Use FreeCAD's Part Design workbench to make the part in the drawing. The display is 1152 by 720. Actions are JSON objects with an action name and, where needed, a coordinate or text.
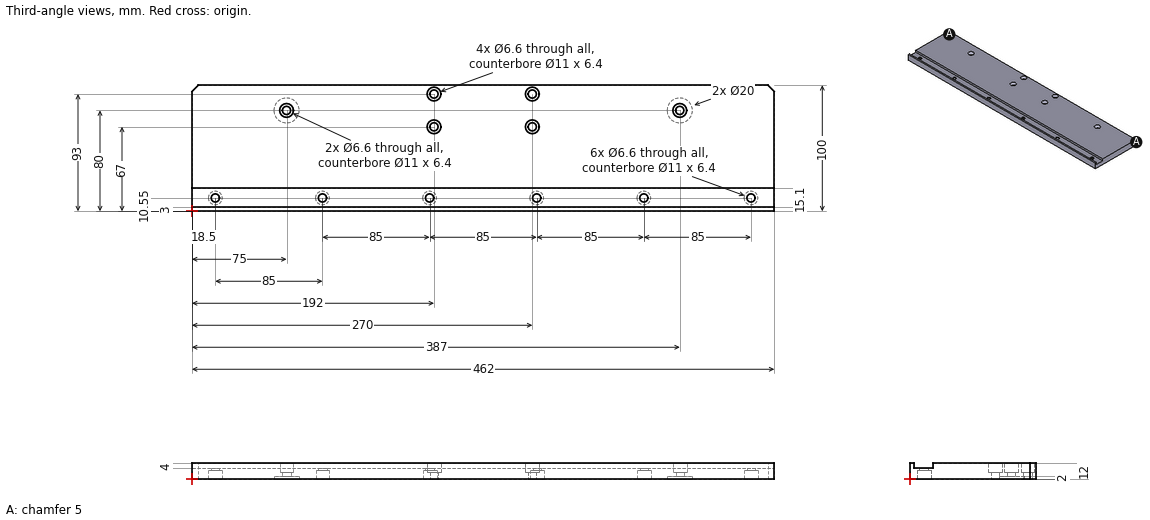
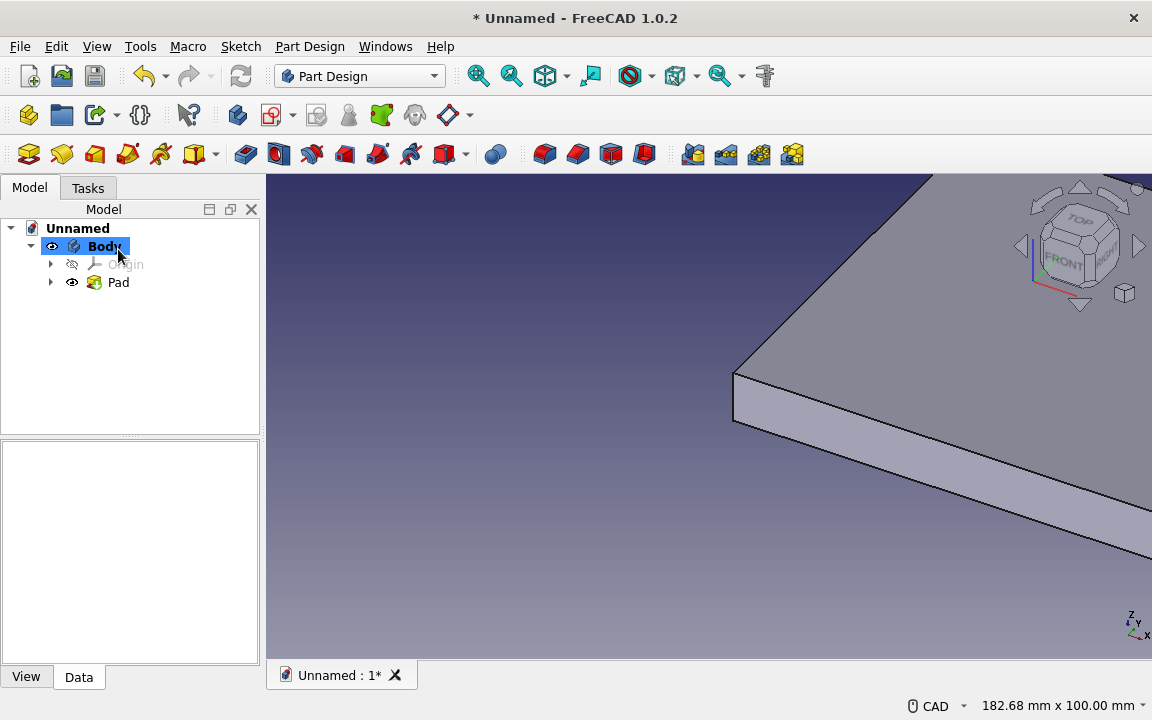
{"action": "key", "text": "v f"}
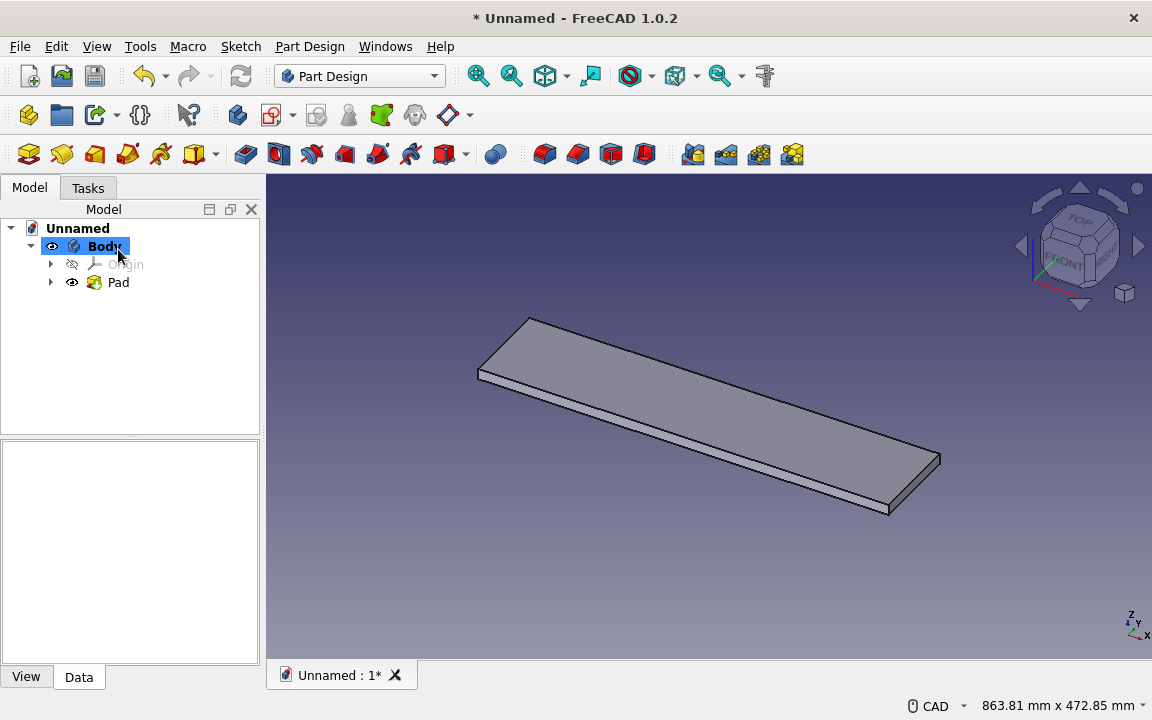
{"action": "left_click", "coordinate": [826, 449]}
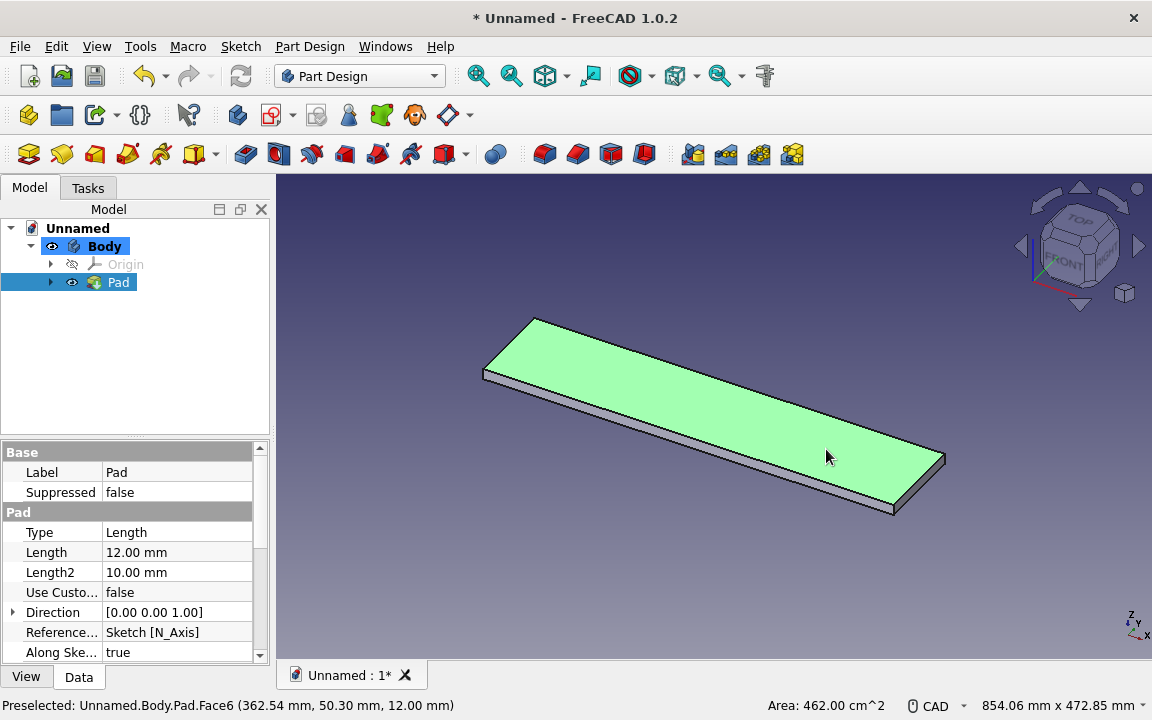
{"action": "left_click", "coordinate": [270, 116]}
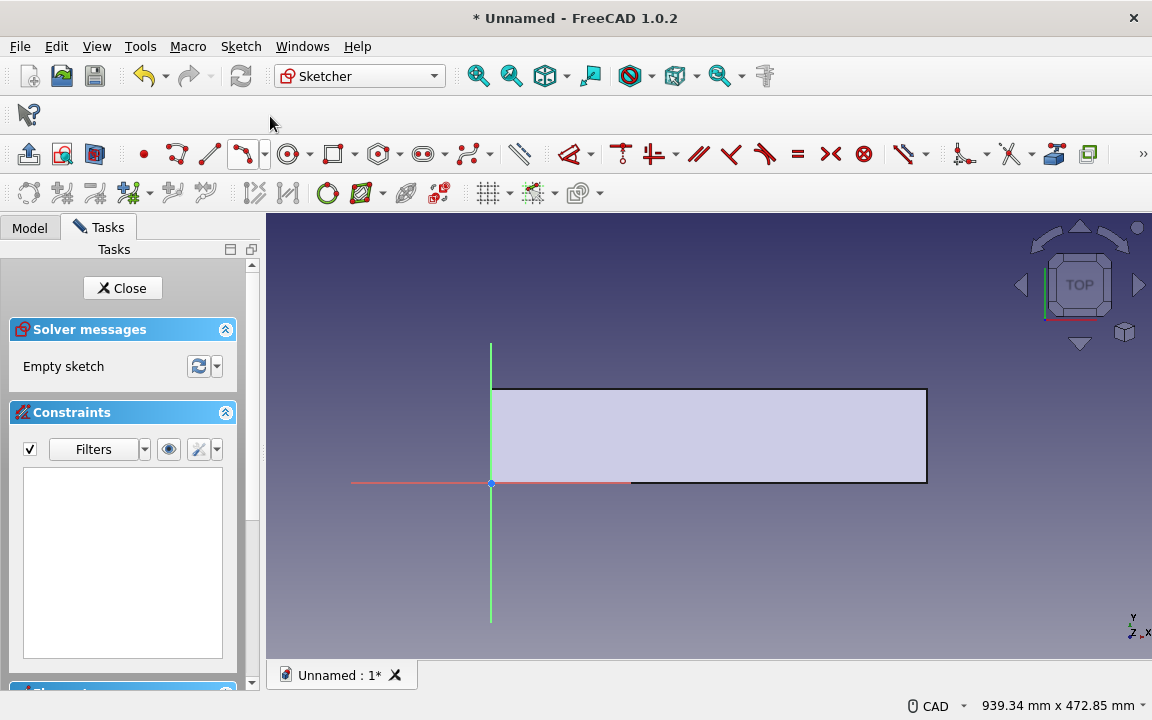
{"action": "left_click", "coordinate": [332, 154]}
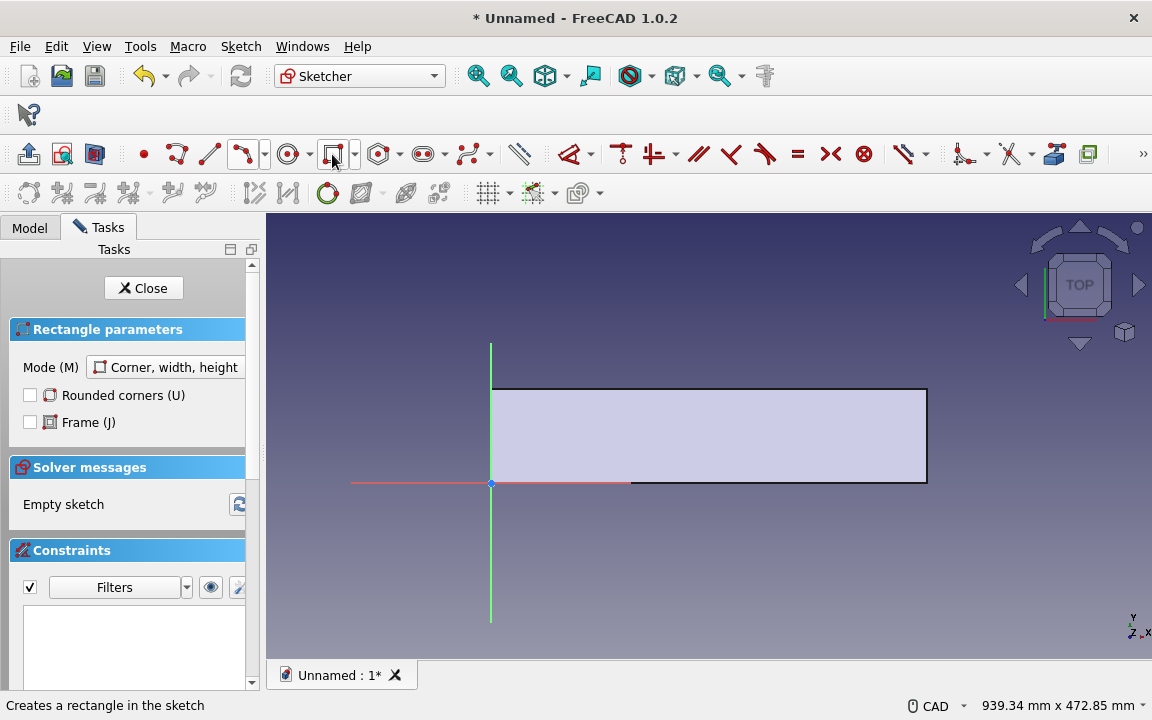
{"action": "left_click", "coordinate": [491, 466]}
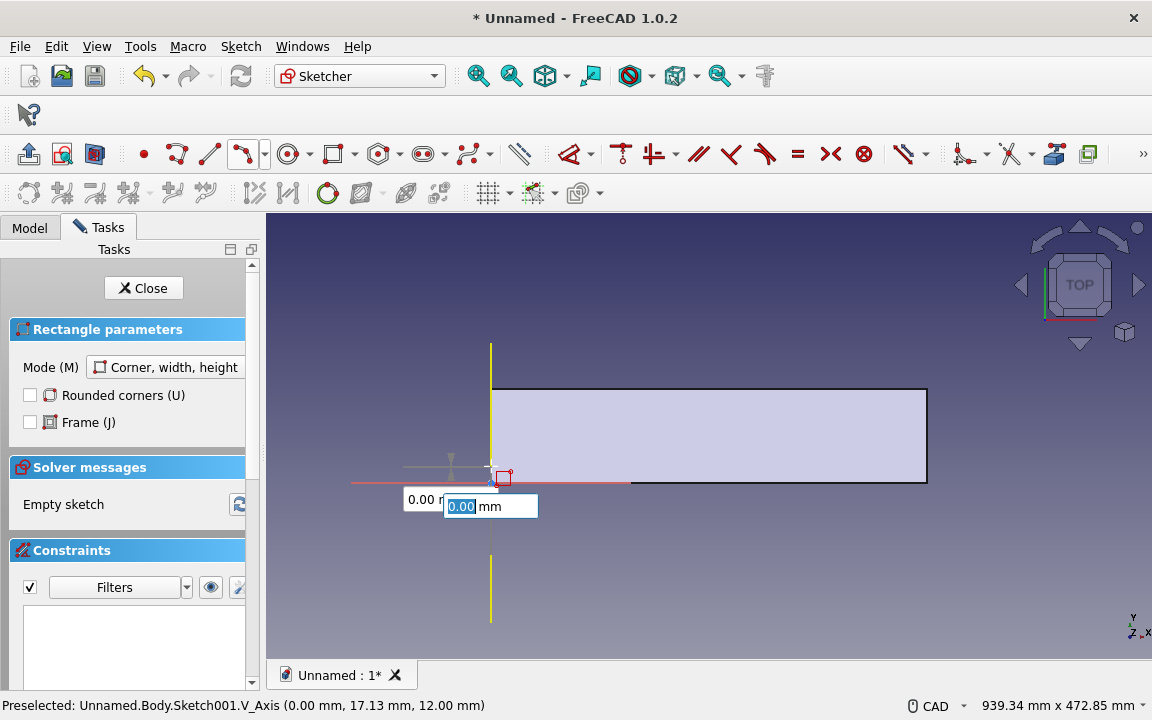
{"action": "scroll", "coordinate": [927, 480], "scroll_direction": "up", "scroll_amount": 9}
{"action": "mouse_move", "coordinate": [923, 479]}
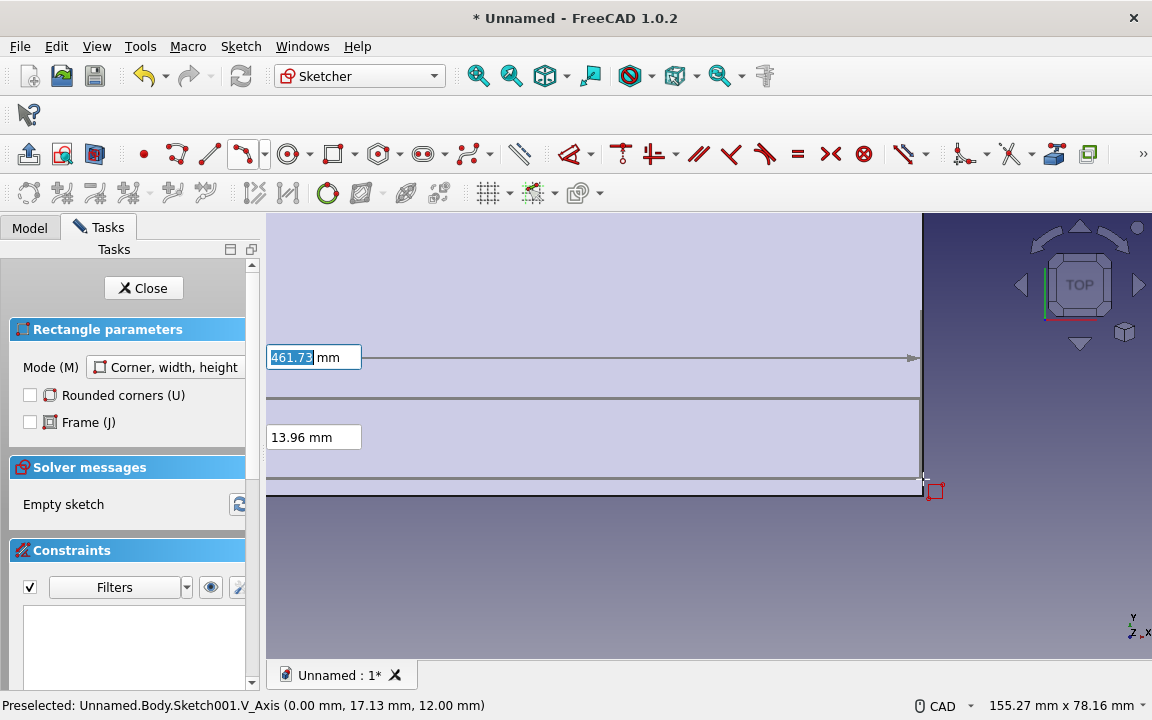
{"action": "type", "text": "462"}
{"action": "key", "text": "Tab"}
{"action": "type", "text": "15.1"}
{"action": "key", "text": "Return"}
{"action": "key", "text": "Escape"}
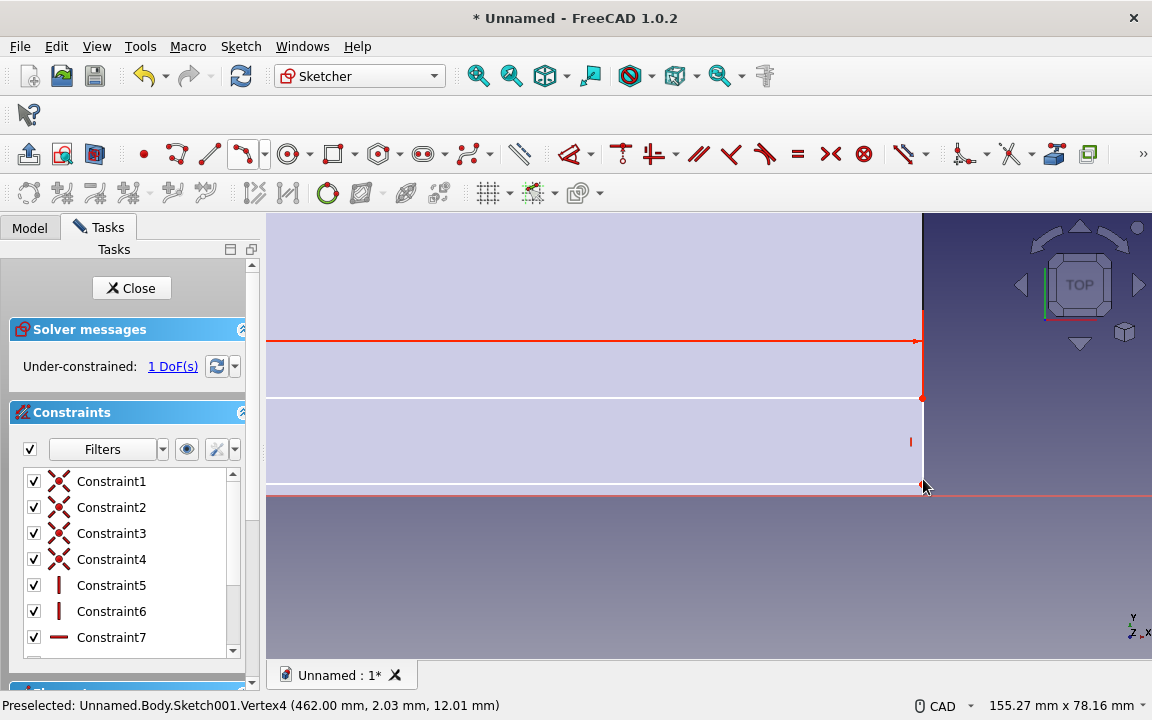
{"action": "left_click", "coordinate": [568, 154]}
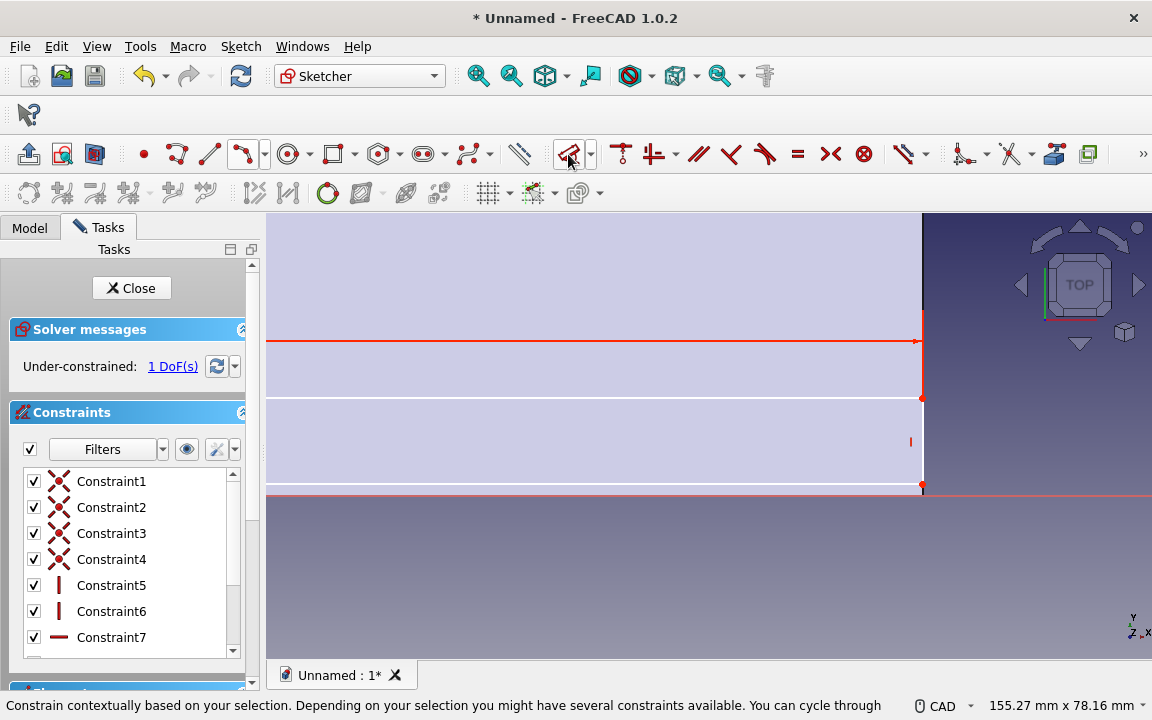
{"action": "scroll", "coordinate": [903, 434], "scroll_direction": "down", "scroll_amount": 8}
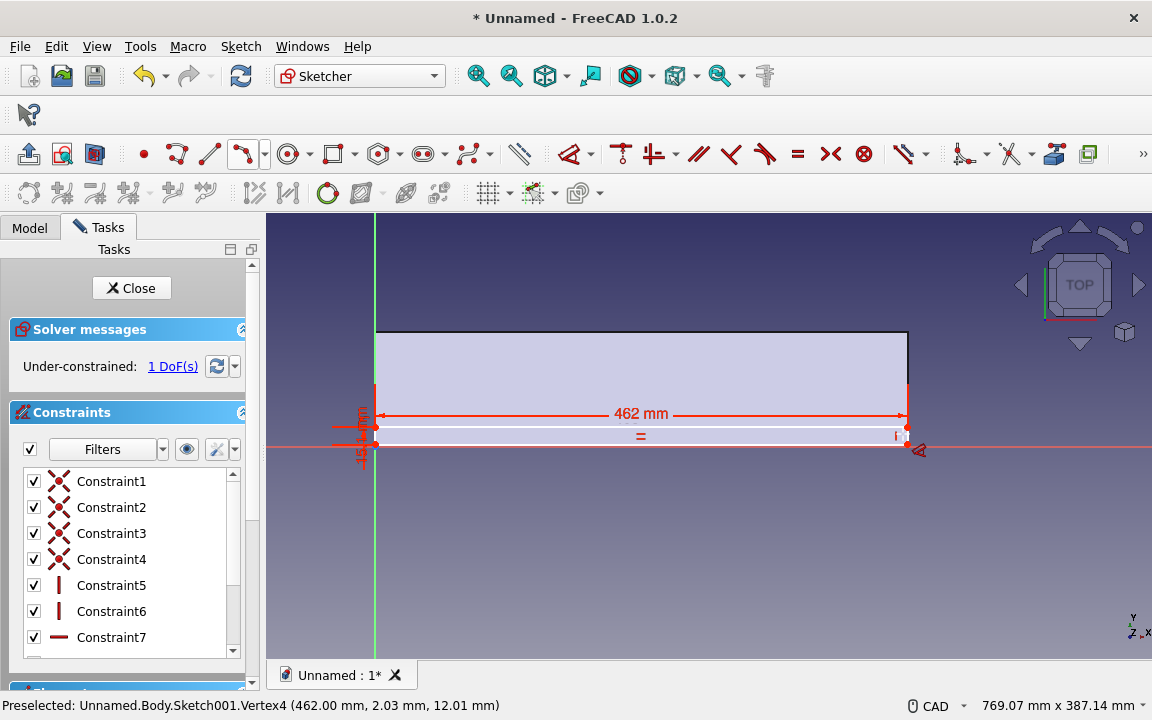
{"action": "scroll", "coordinate": [375, 445], "scroll_direction": "up", "scroll_amount": 13}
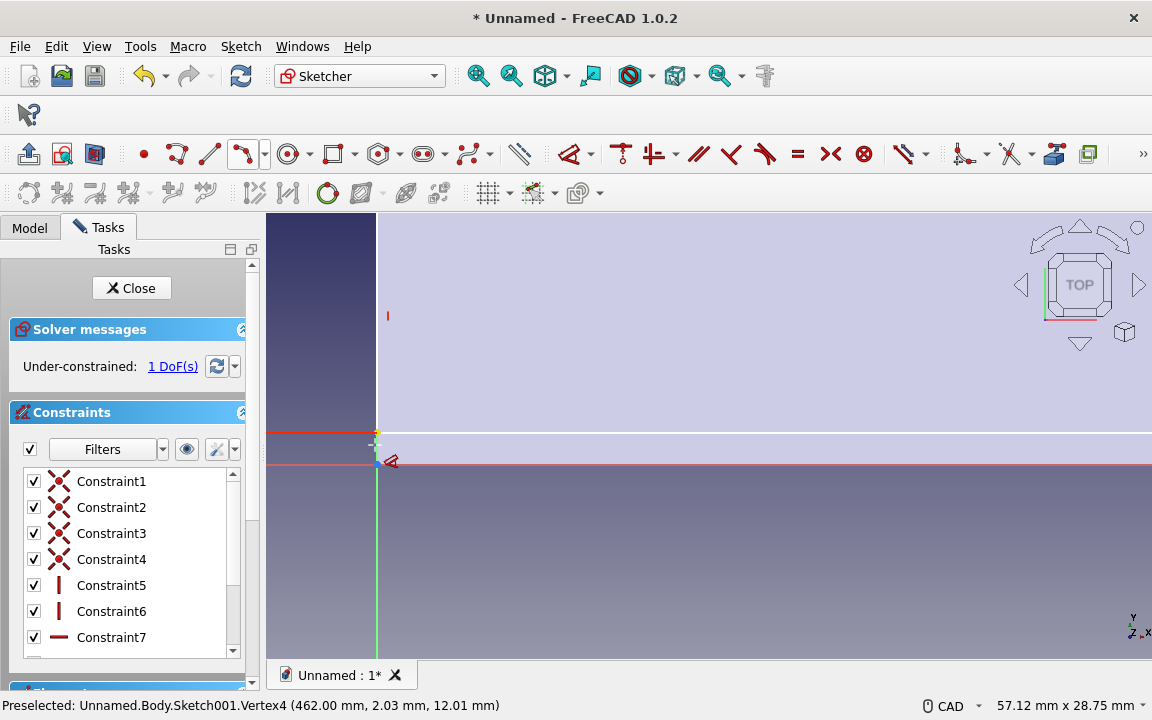
{"action": "left_click", "coordinate": [377, 433]}
{"action": "left_click", "coordinate": [343, 449]}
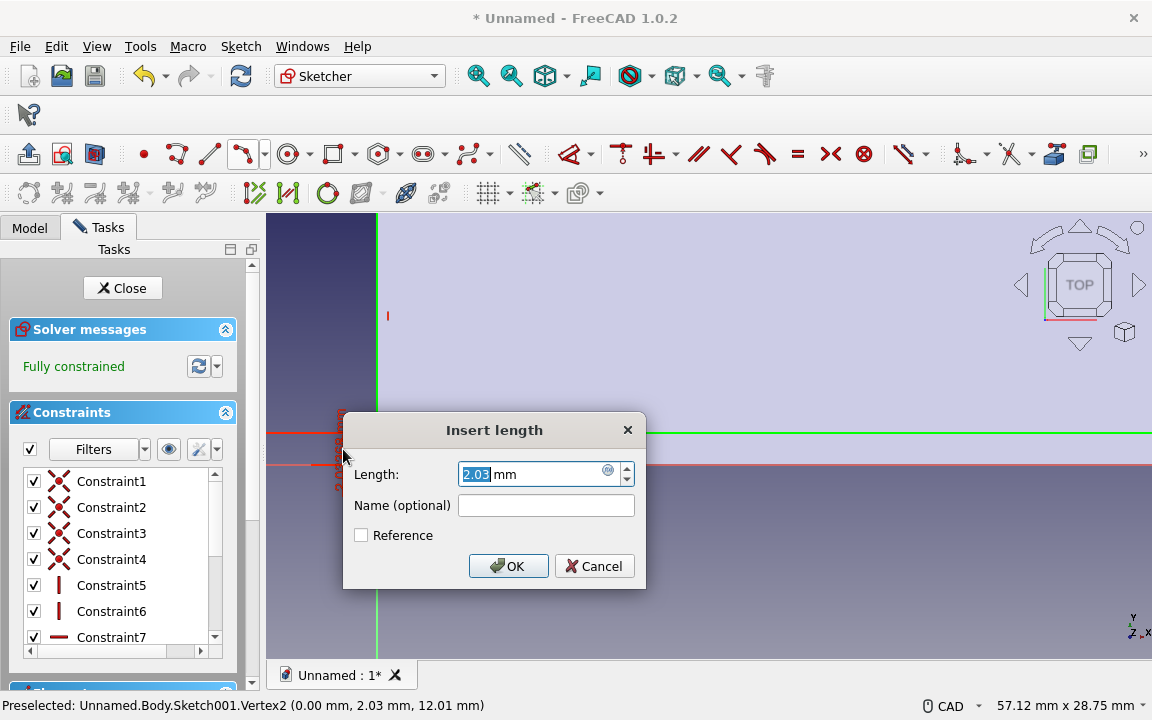
{"action": "type", "text": "3"}
{"action": "key", "text": "Return"}
{"action": "key", "text": "Escape"}